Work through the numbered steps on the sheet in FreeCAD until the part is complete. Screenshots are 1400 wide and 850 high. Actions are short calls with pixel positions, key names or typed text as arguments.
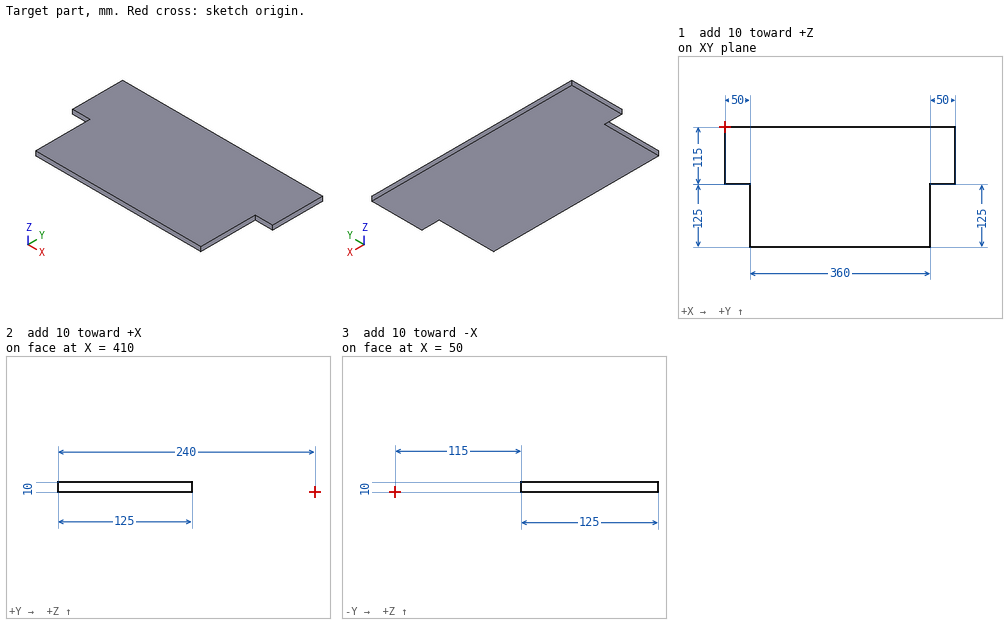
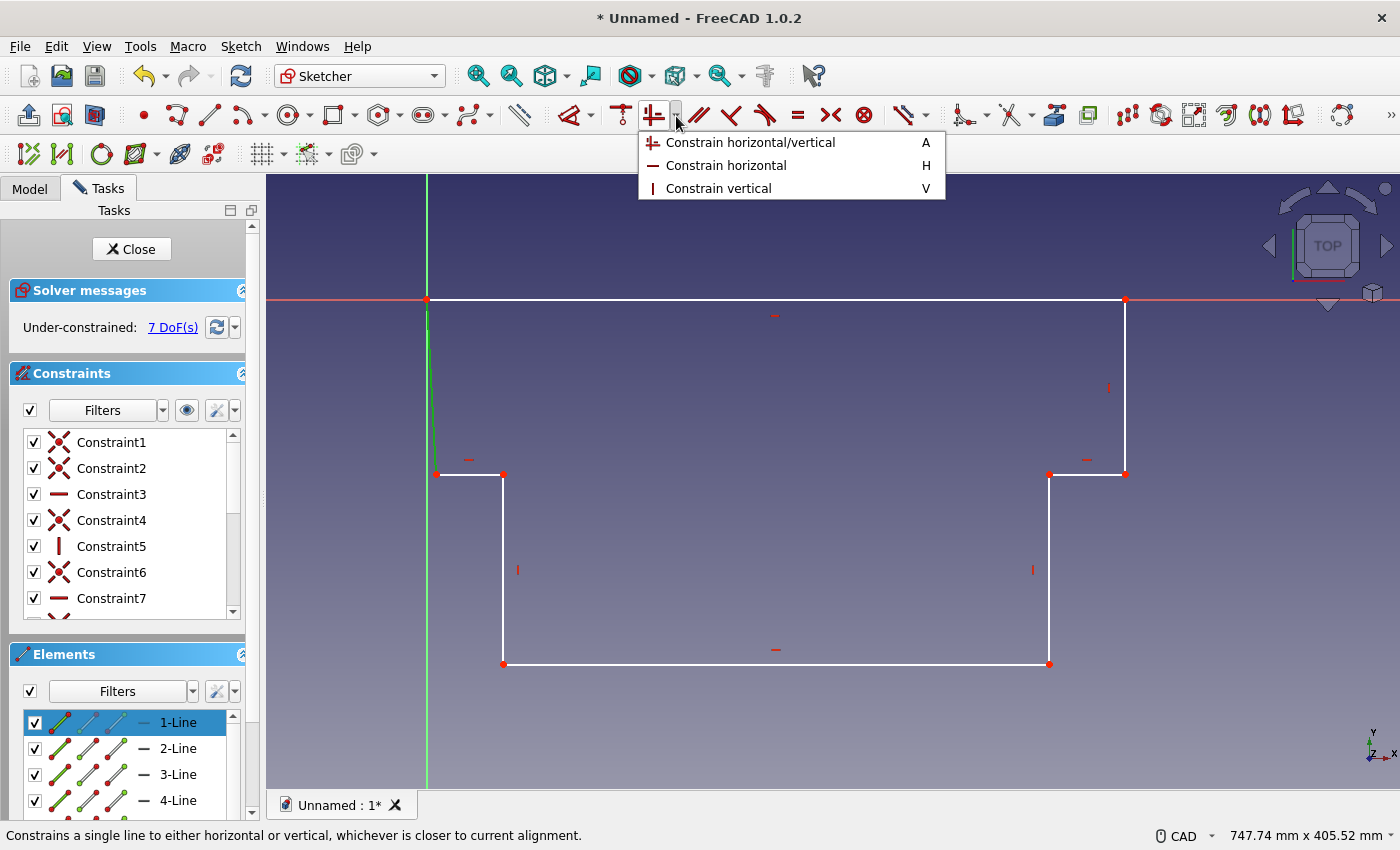
click(792, 188)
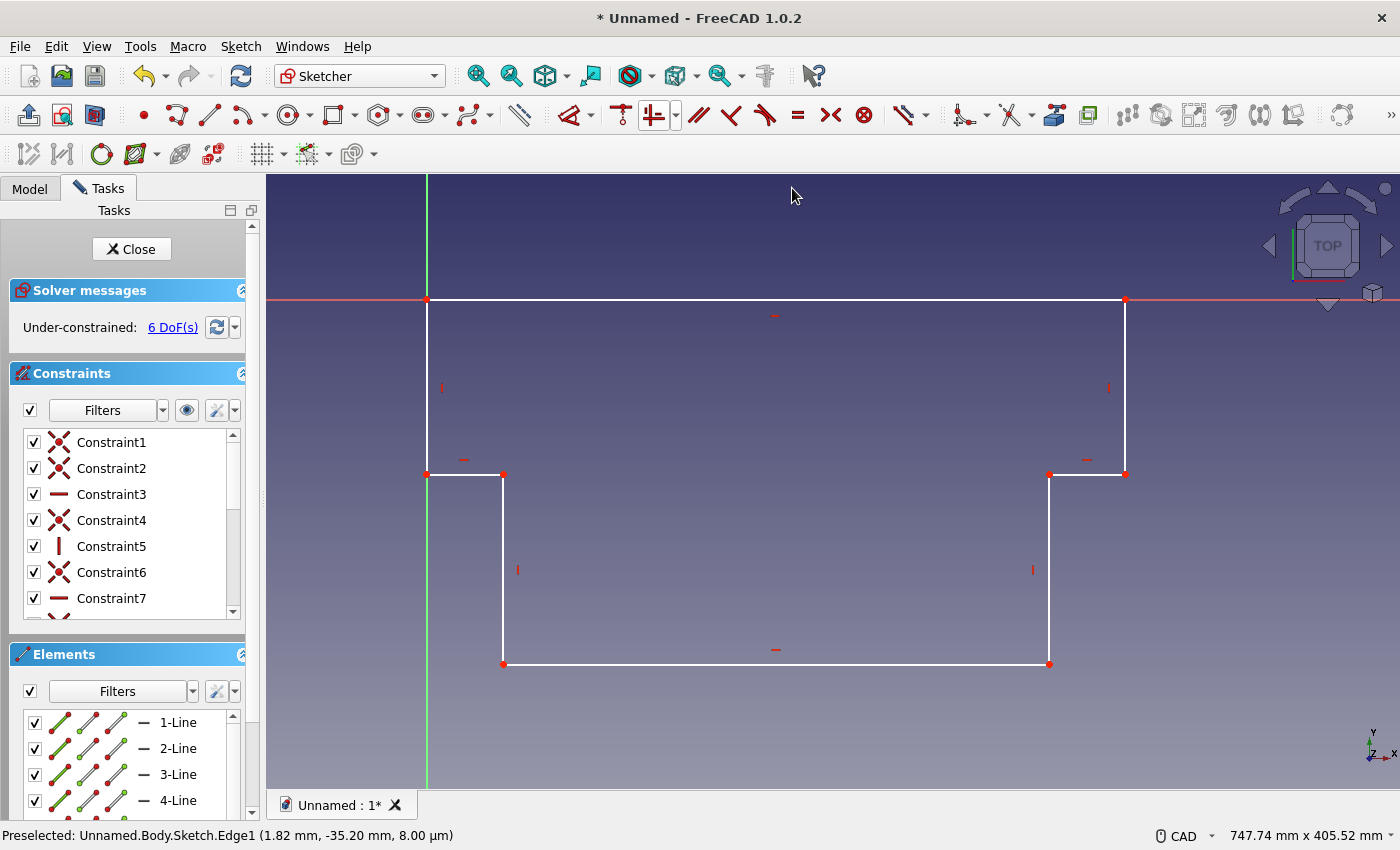
click(450, 475)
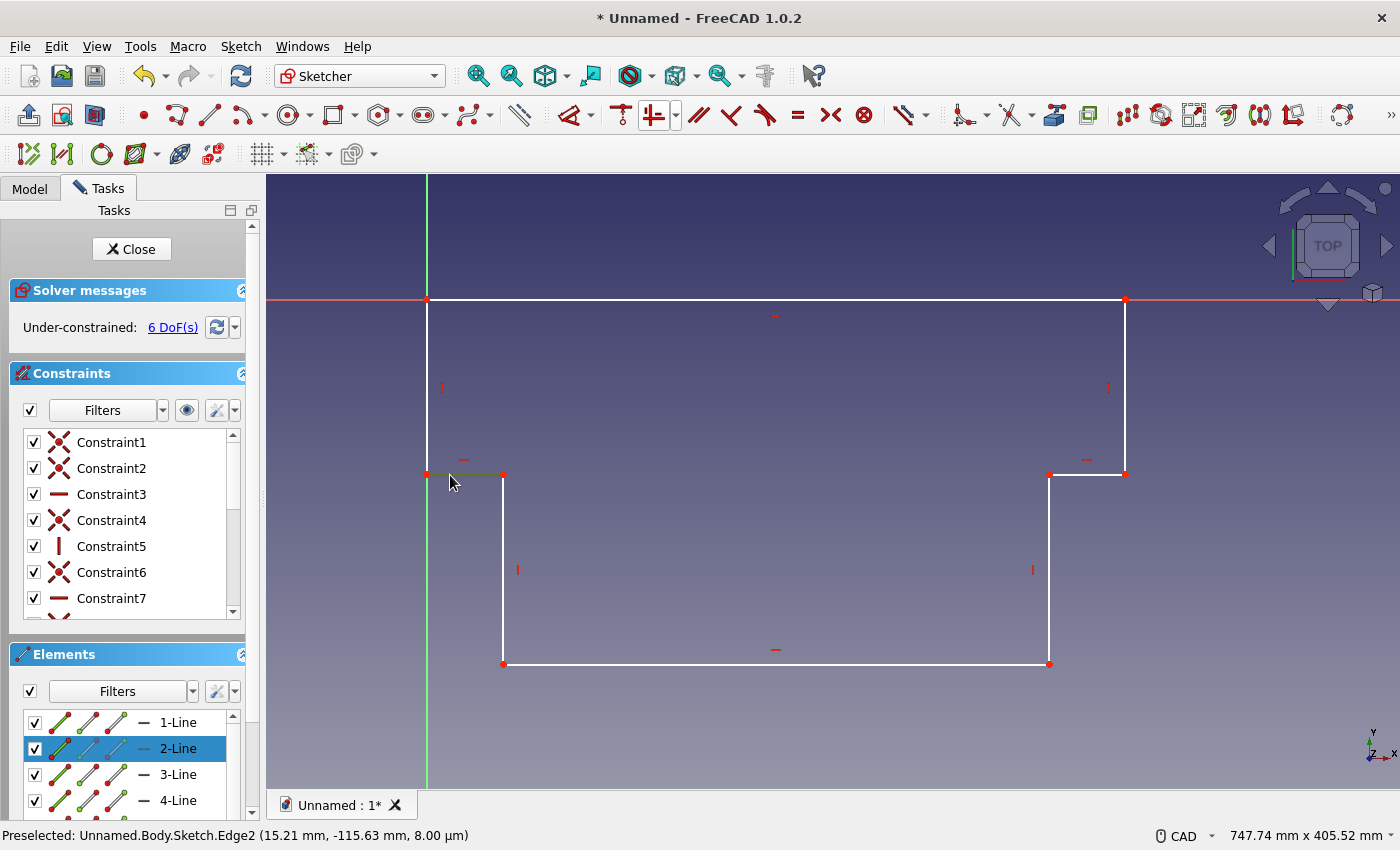
click(590, 116)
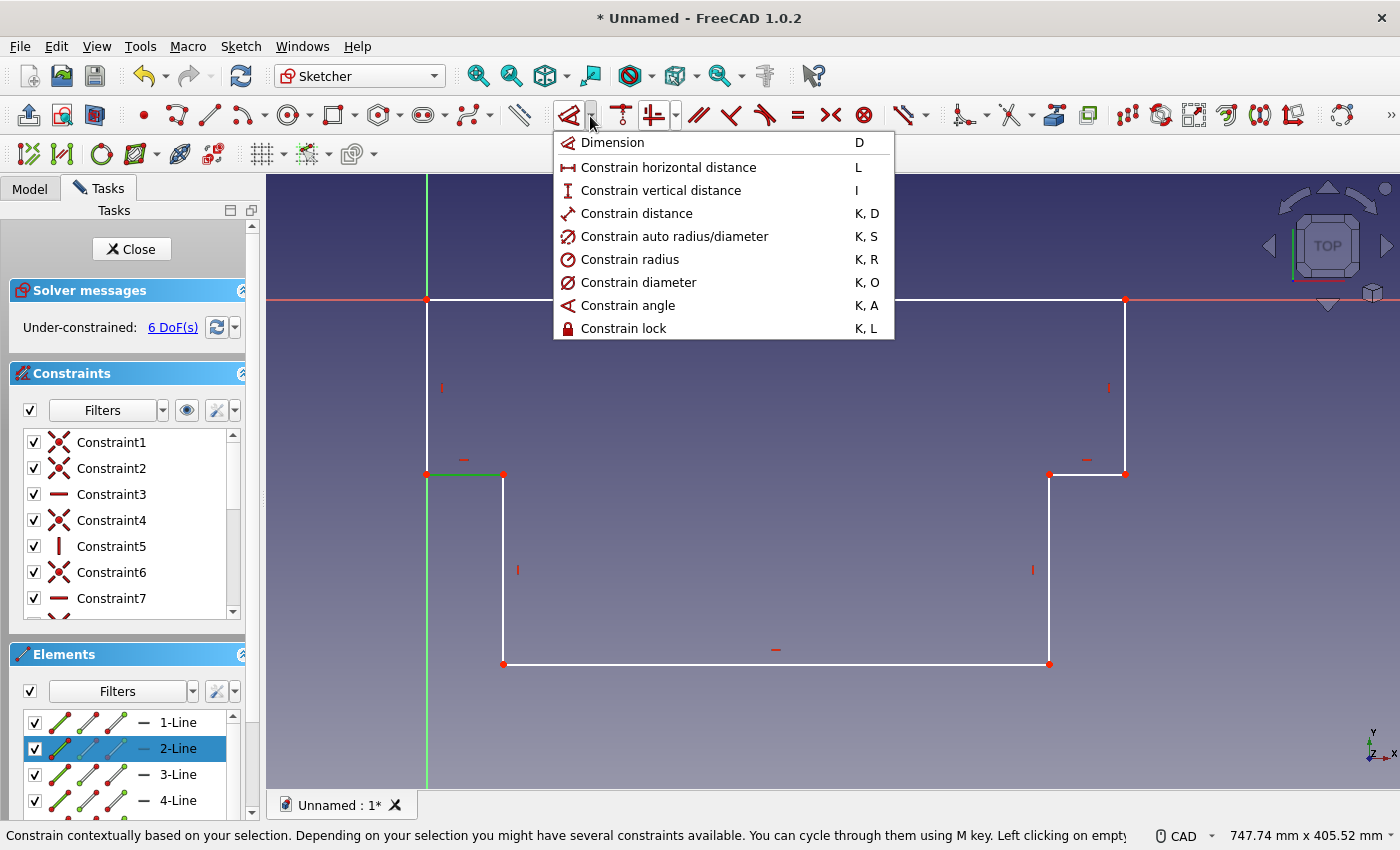
click(724, 168)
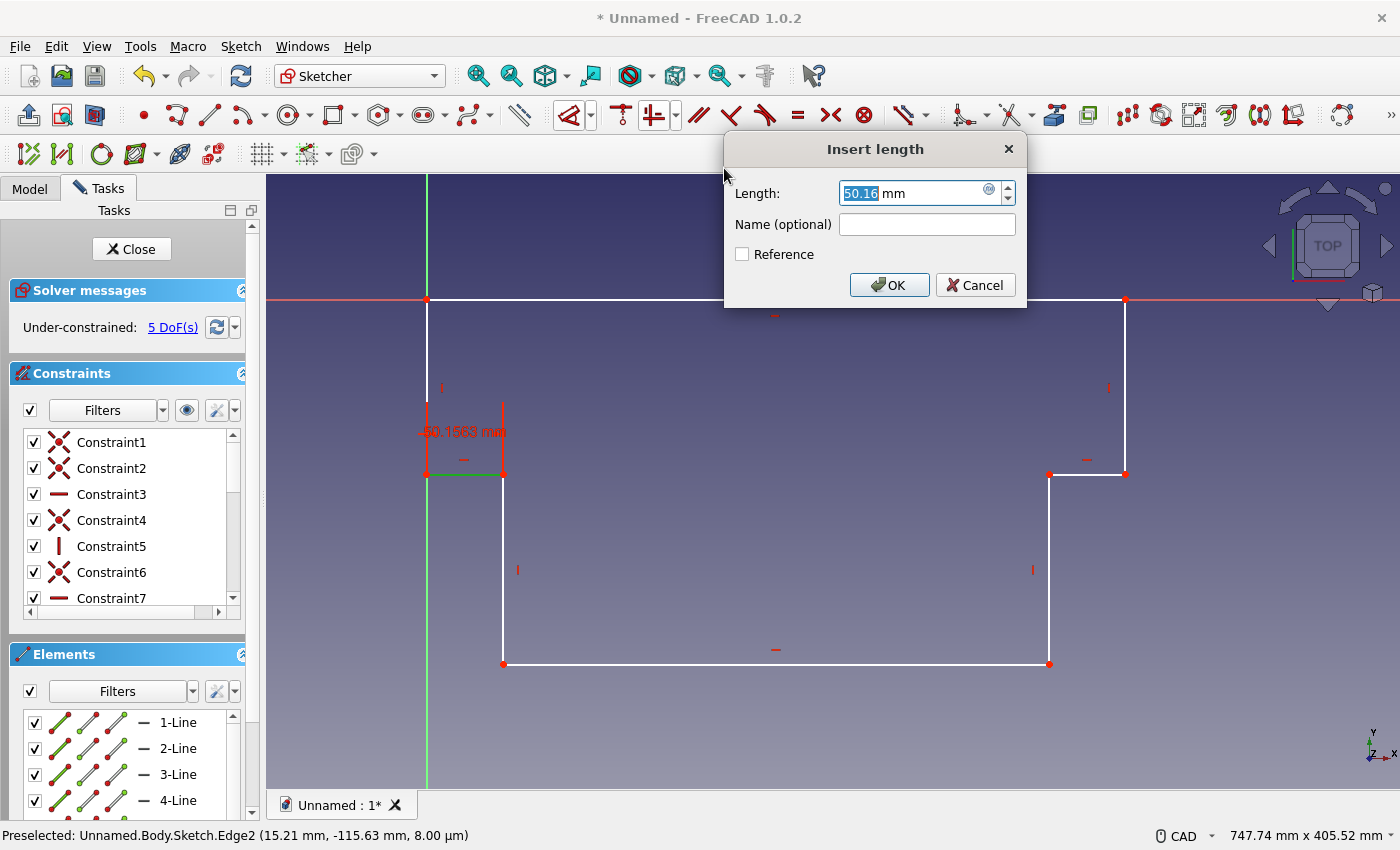
text(50)
key(Return)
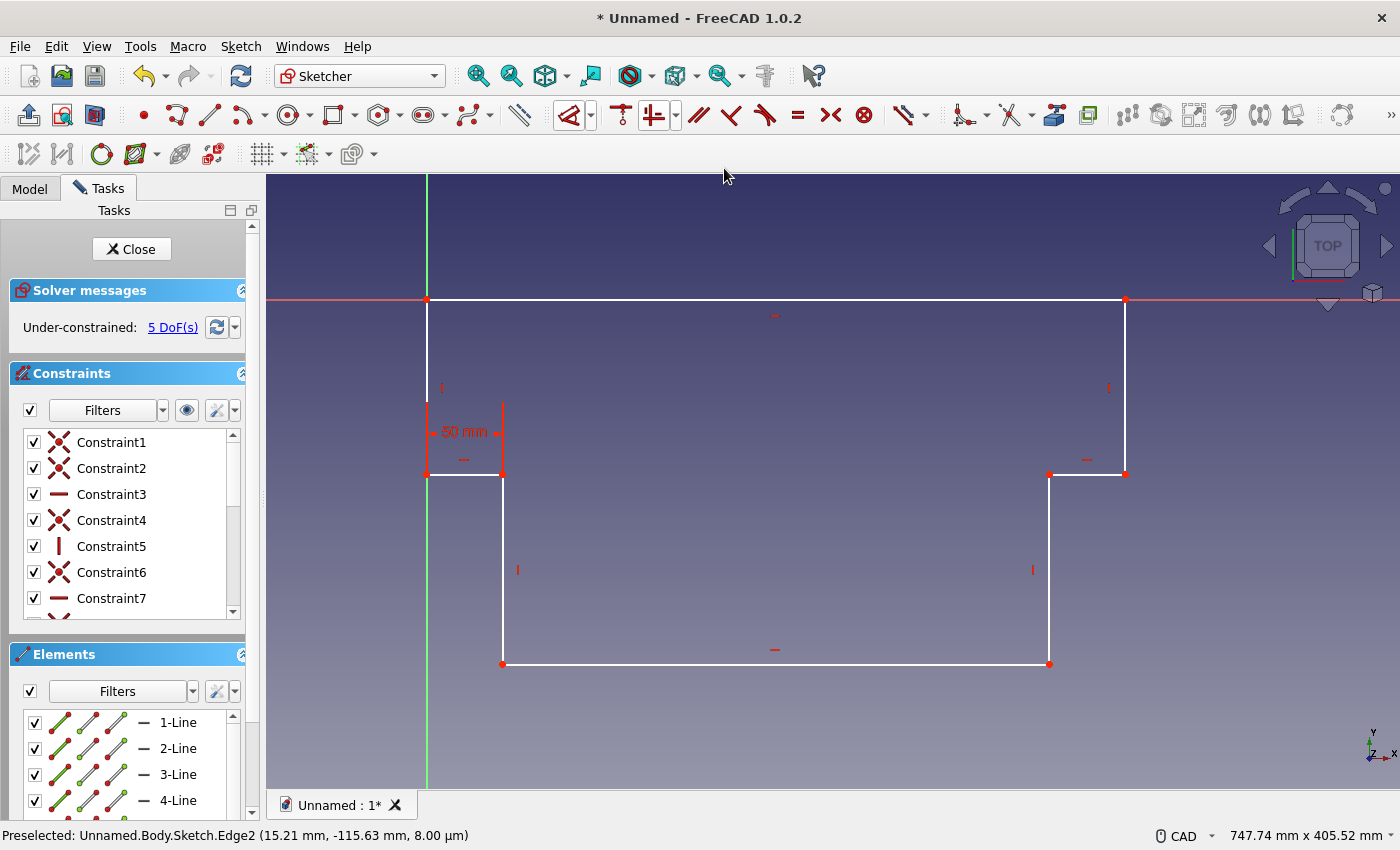
click(1072, 475)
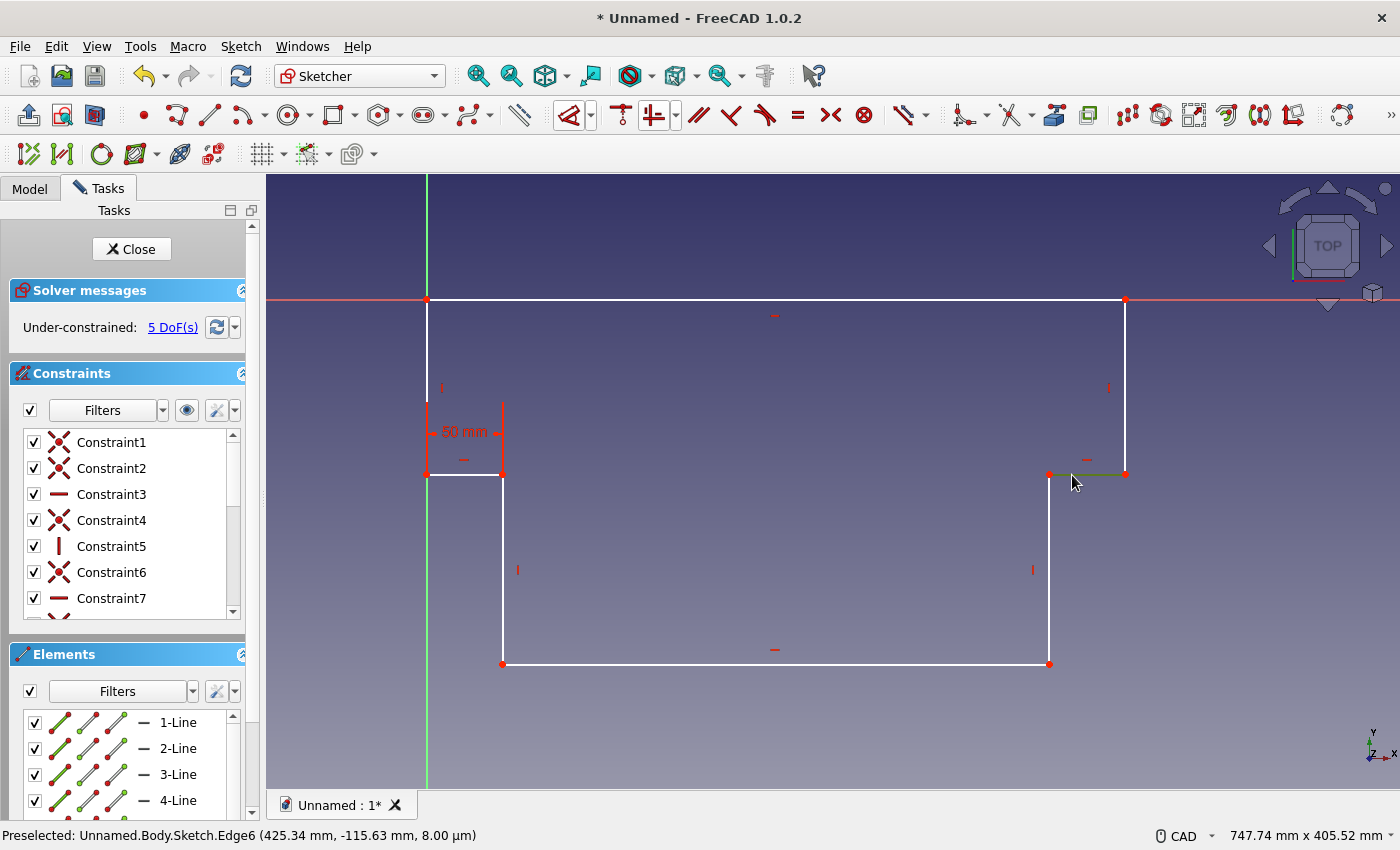
key(l)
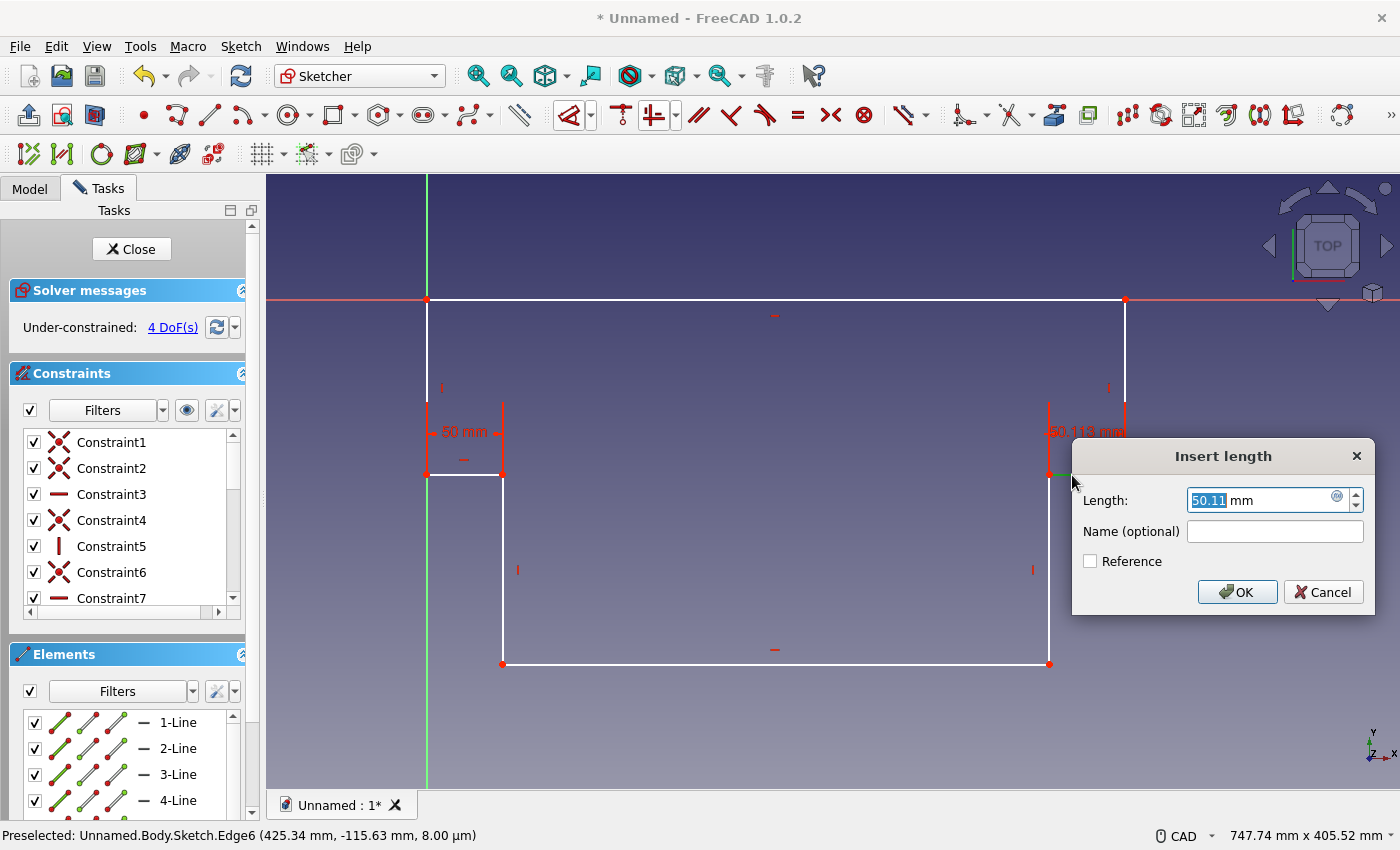
text(50)
key(Return)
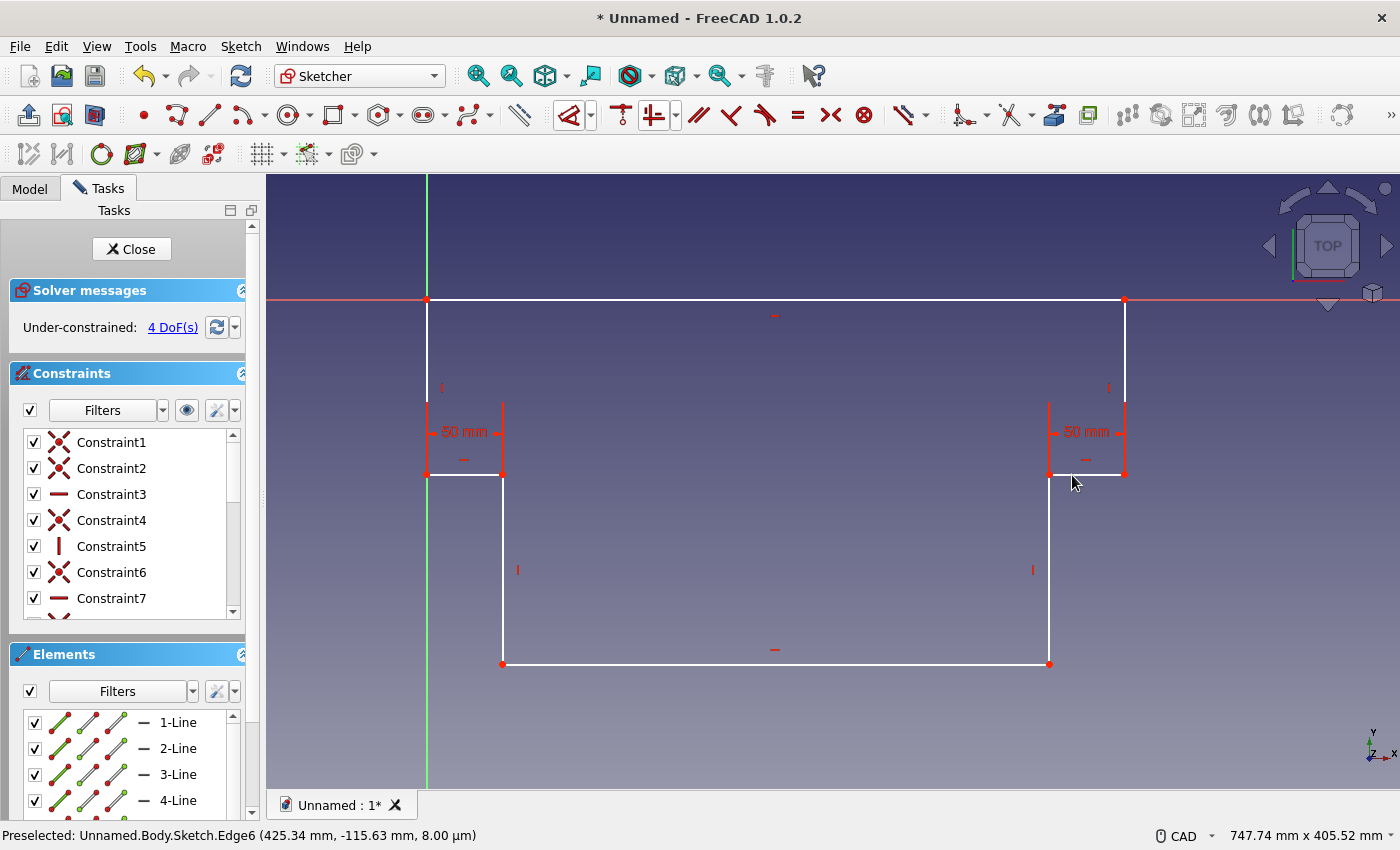
click(427, 352)